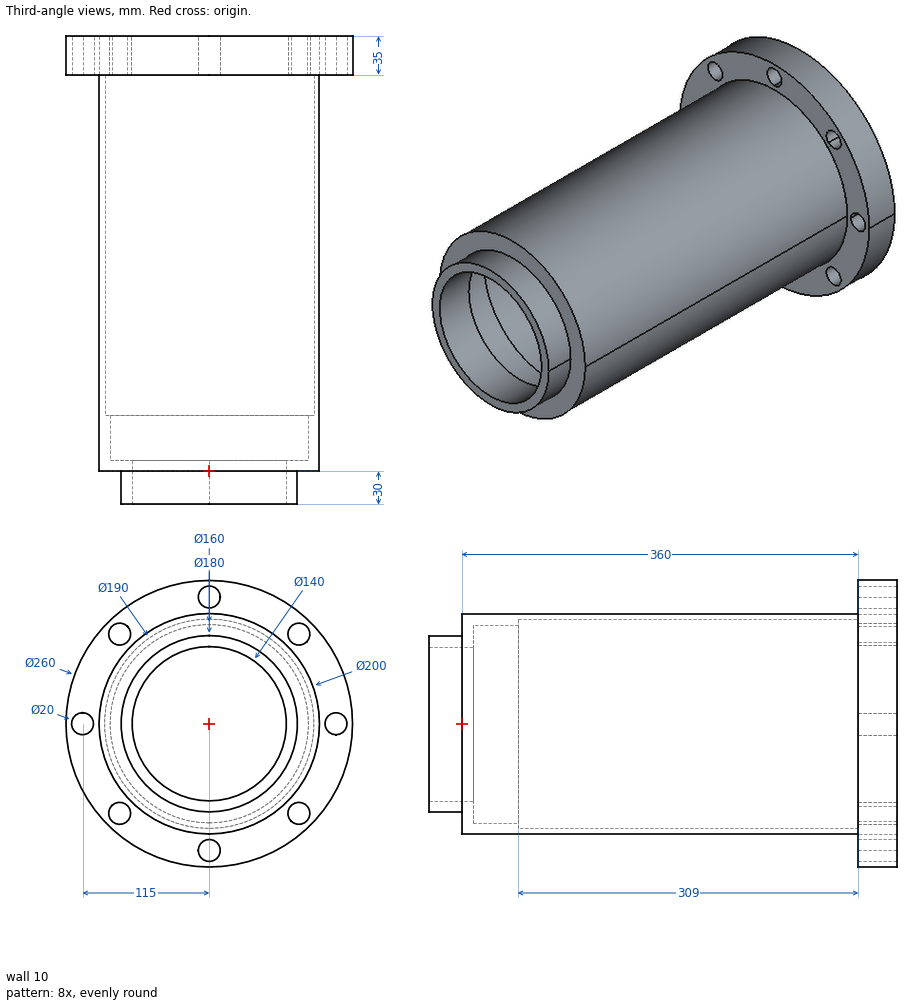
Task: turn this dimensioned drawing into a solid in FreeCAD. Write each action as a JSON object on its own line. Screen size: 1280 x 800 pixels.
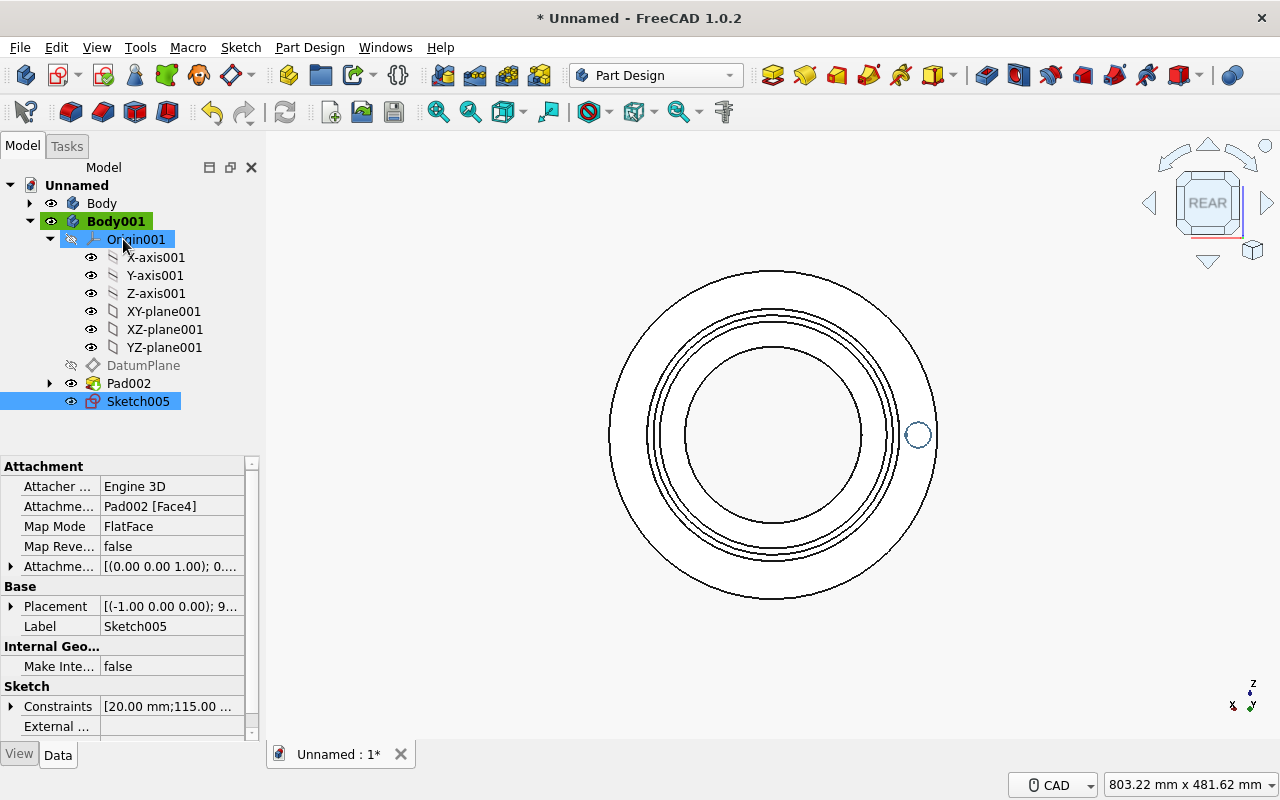
{"action": "left_click", "coordinate": [988, 76]}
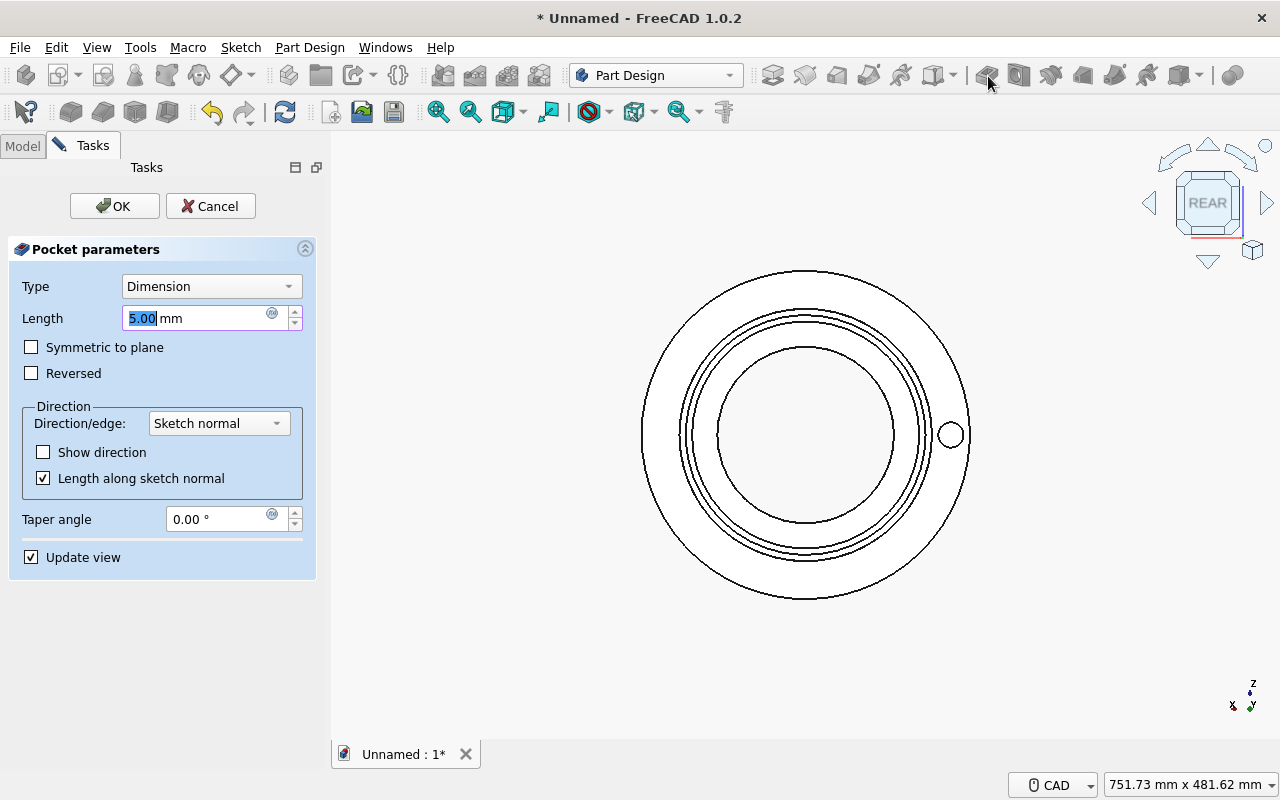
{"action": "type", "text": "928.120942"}
{"action": "key", "text": "Tab"}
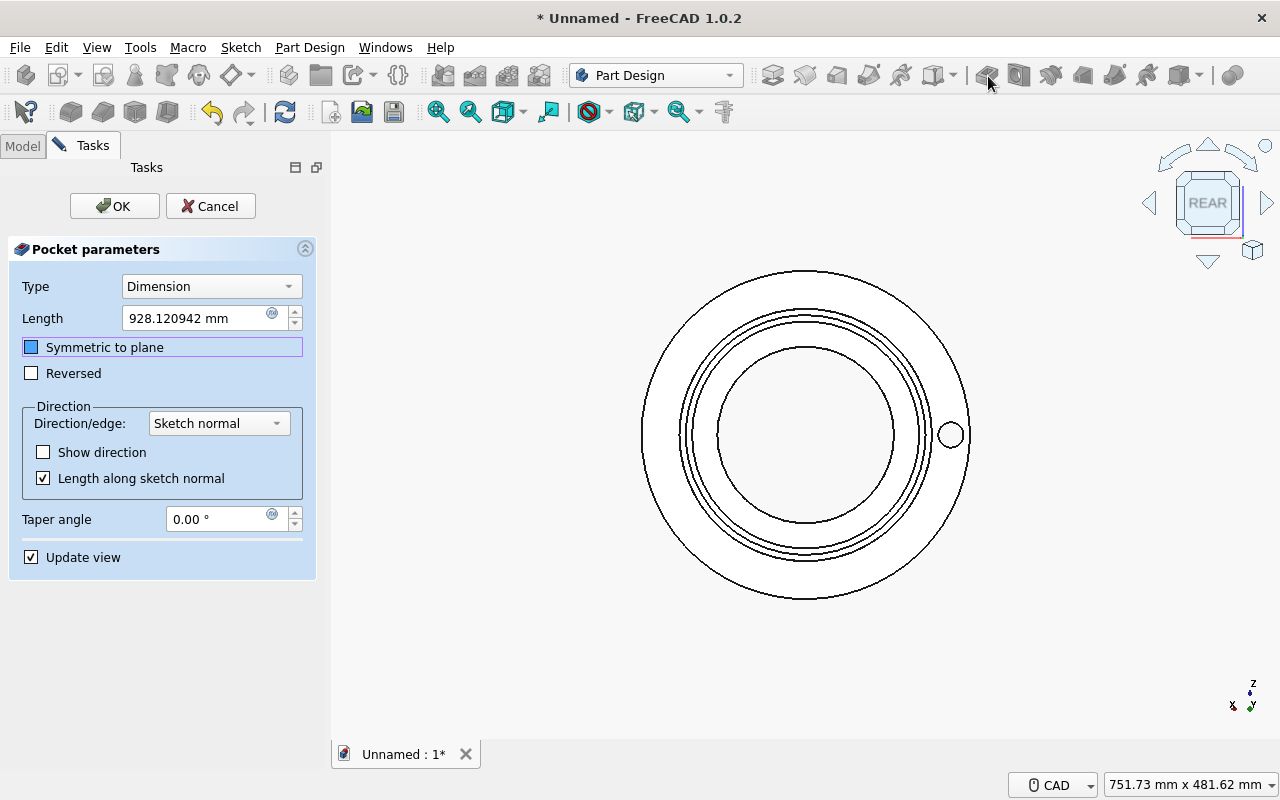
{"action": "left_click", "coordinate": [30, 347]}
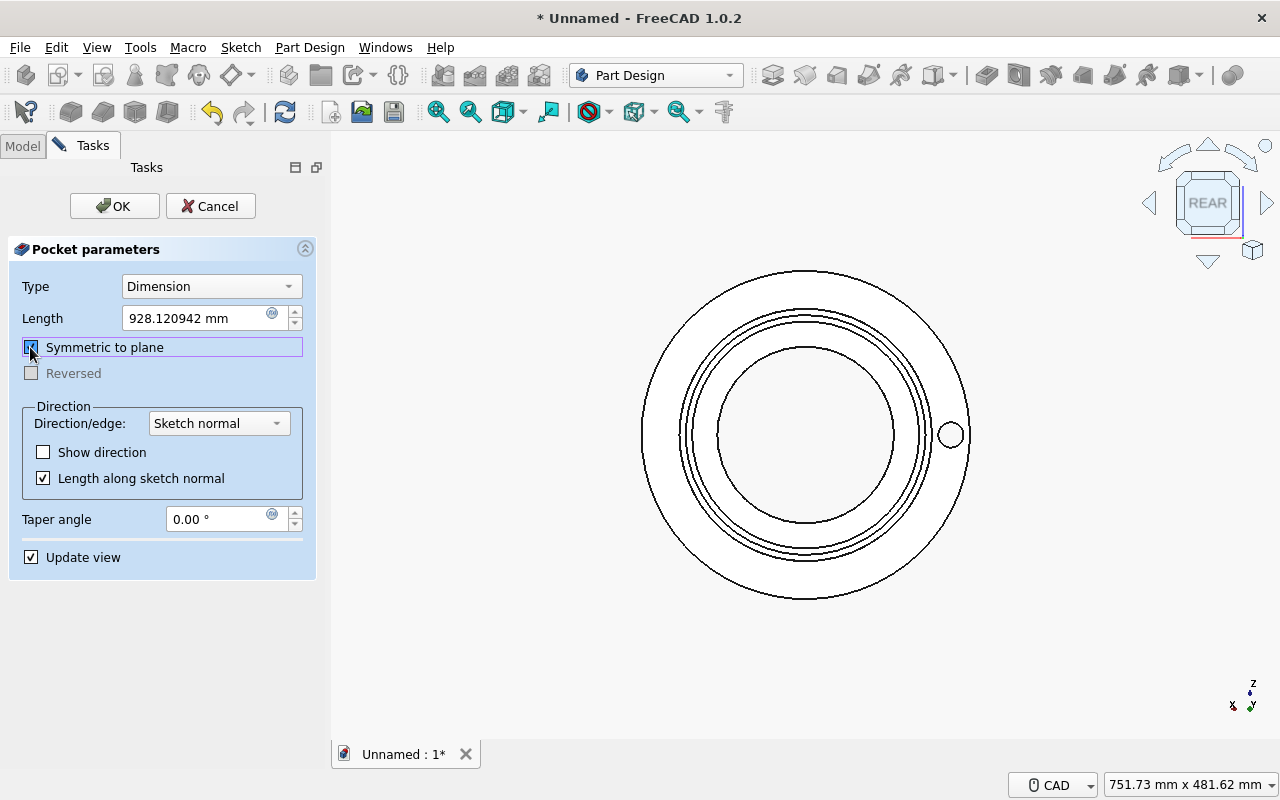
{"action": "left_click", "coordinate": [115, 206]}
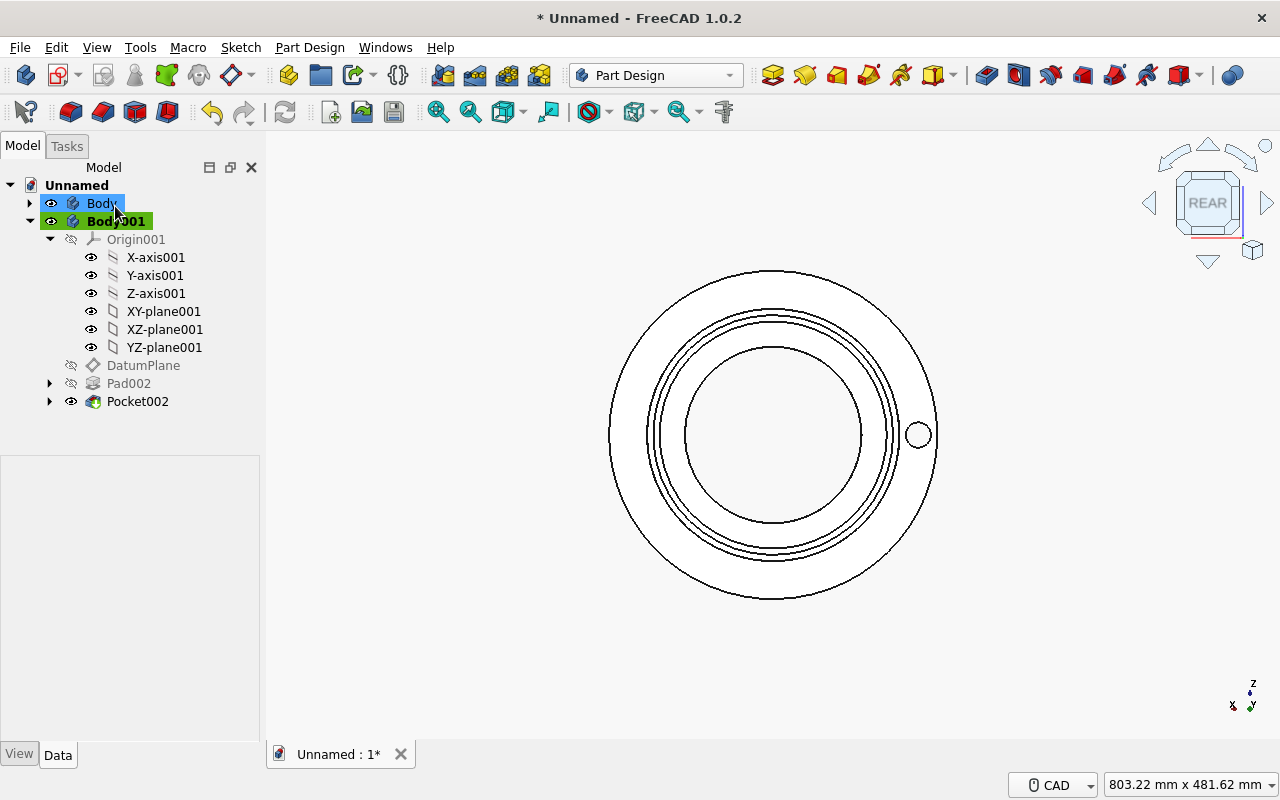
{"action": "left_click", "coordinate": [116, 401]}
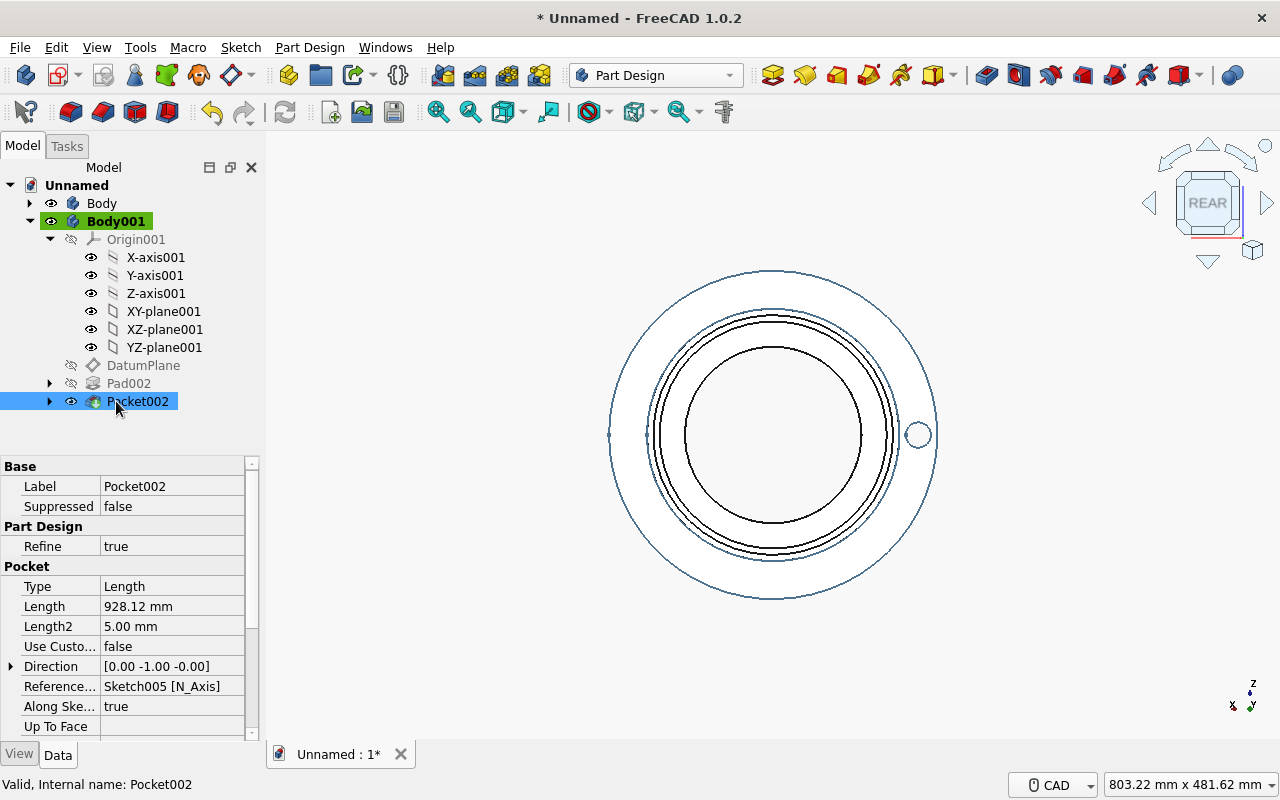
{"action": "left_click", "coordinate": [508, 76]}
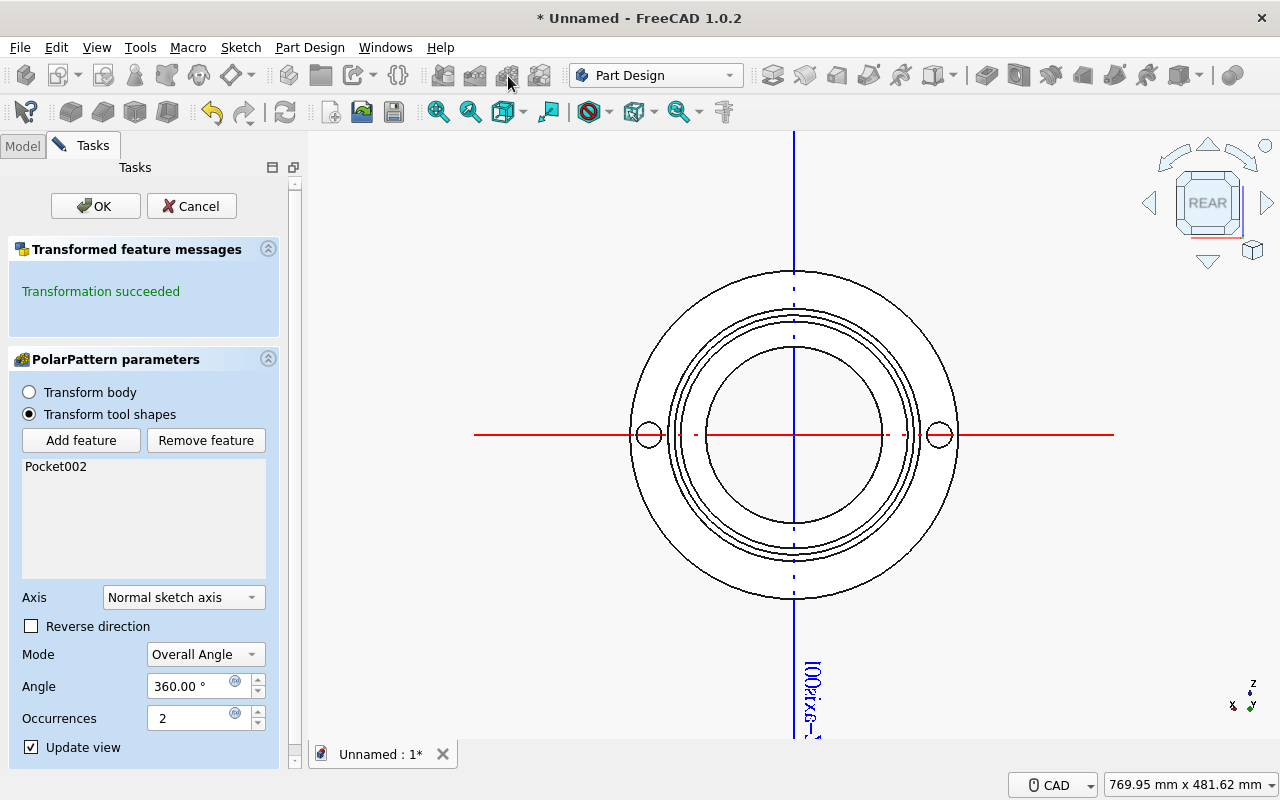
{"action": "left_click", "coordinate": [184, 598]}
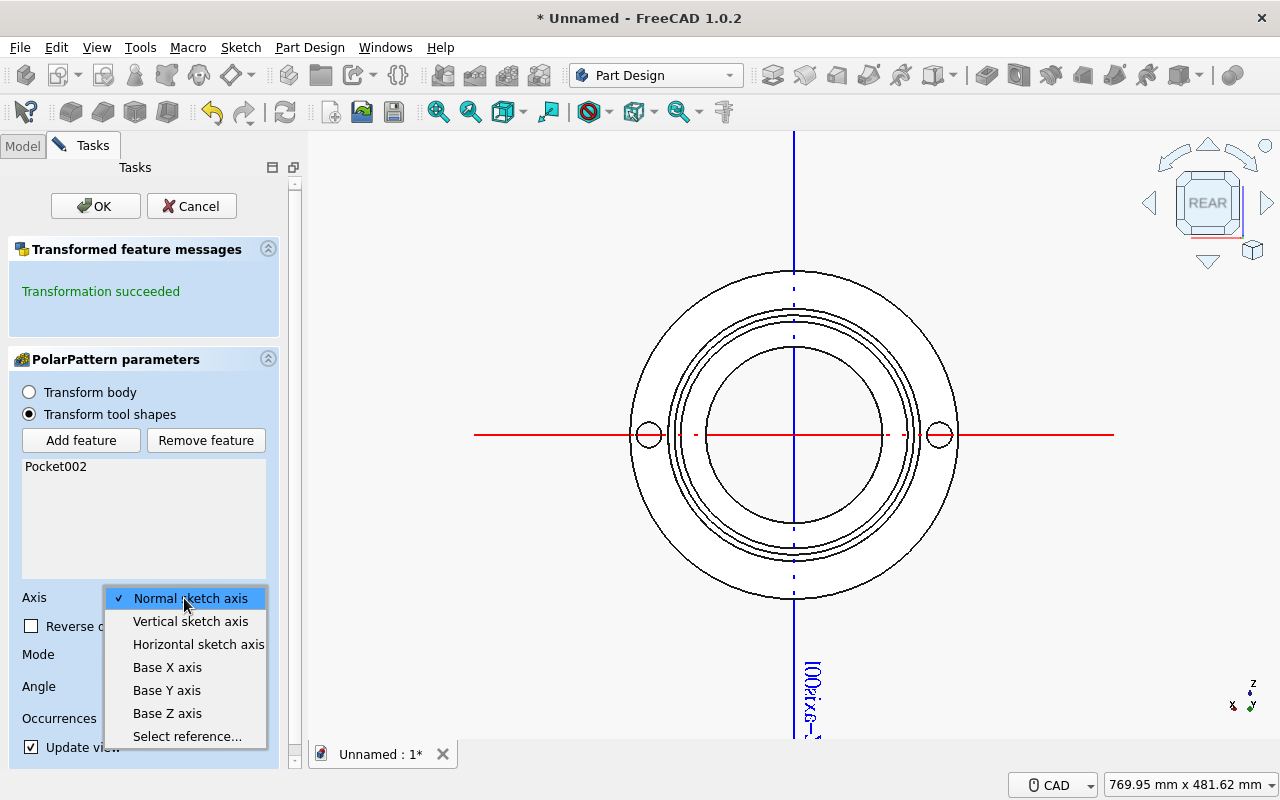
{"action": "left_click", "coordinate": [184, 690]}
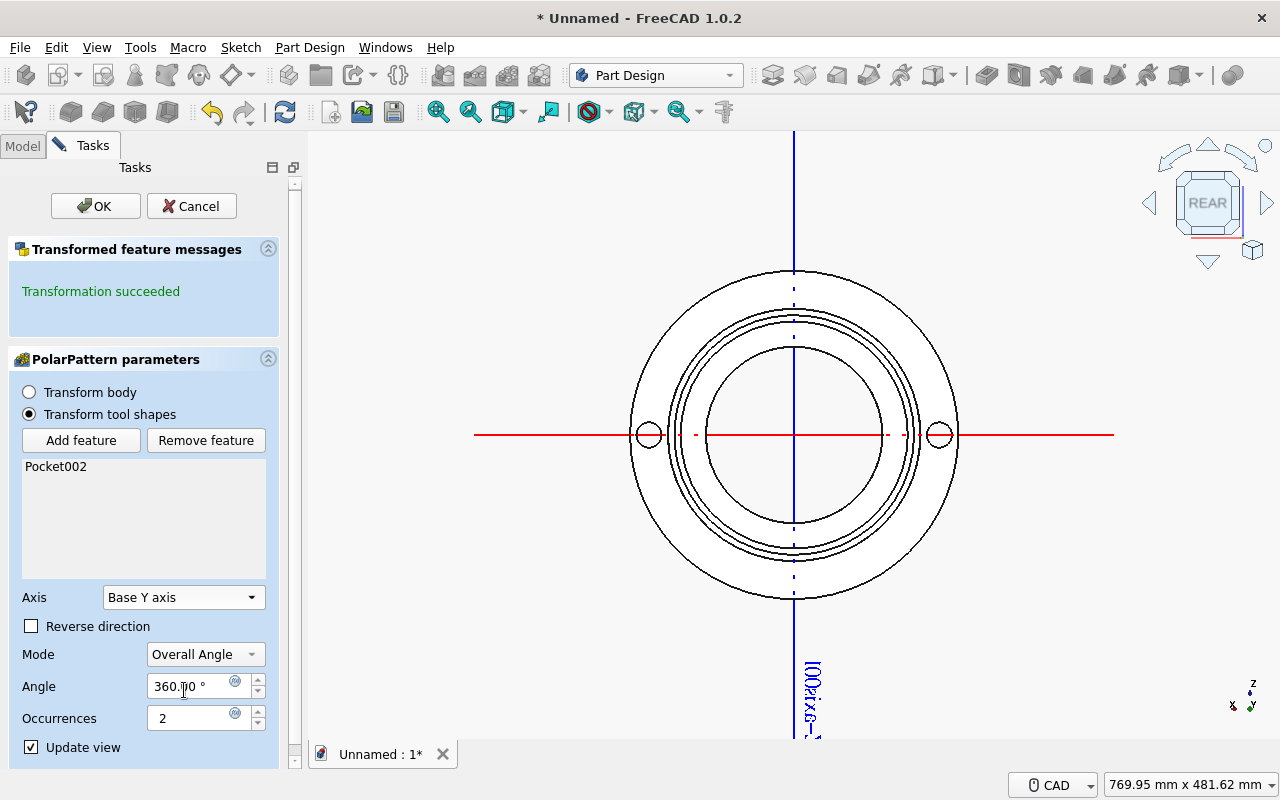
{"action": "triple_click", "coordinate": [198, 718]}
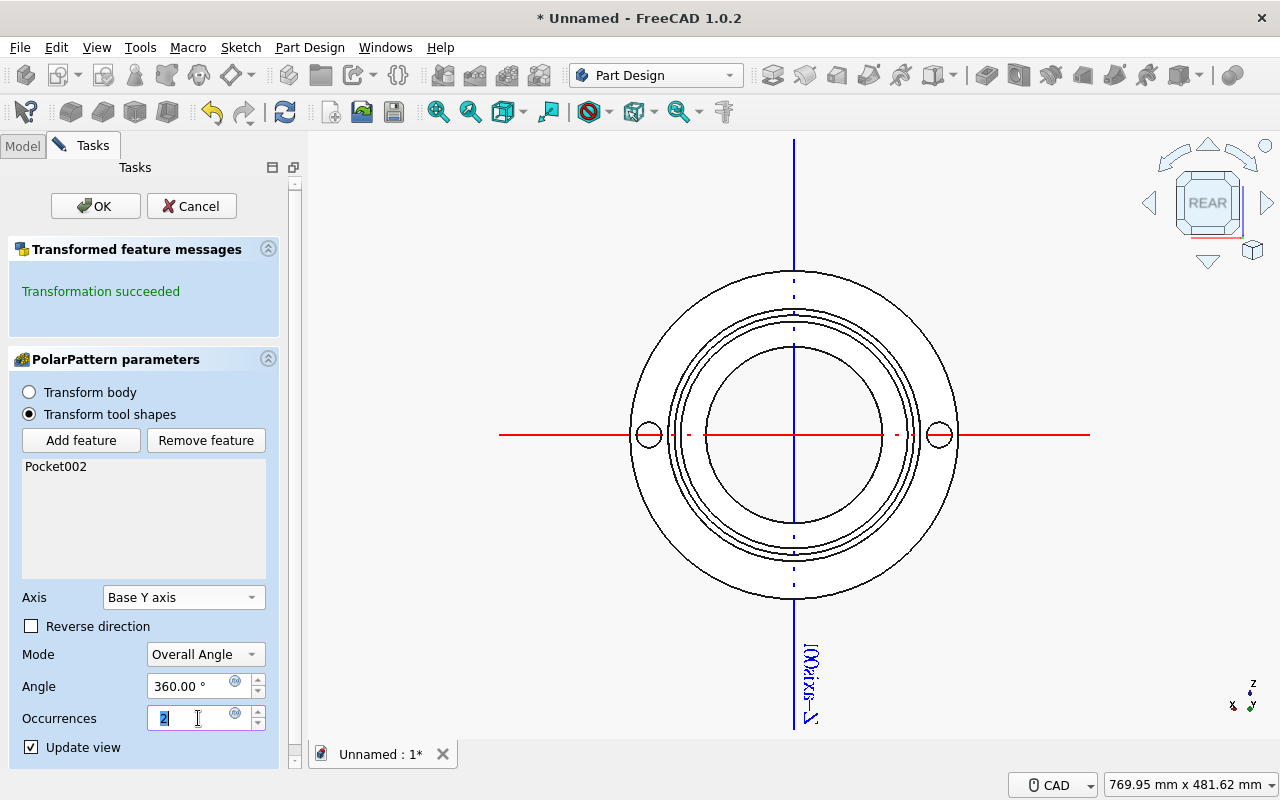
{"action": "type", "text": "8"}
{"action": "key", "text": "Tab"}